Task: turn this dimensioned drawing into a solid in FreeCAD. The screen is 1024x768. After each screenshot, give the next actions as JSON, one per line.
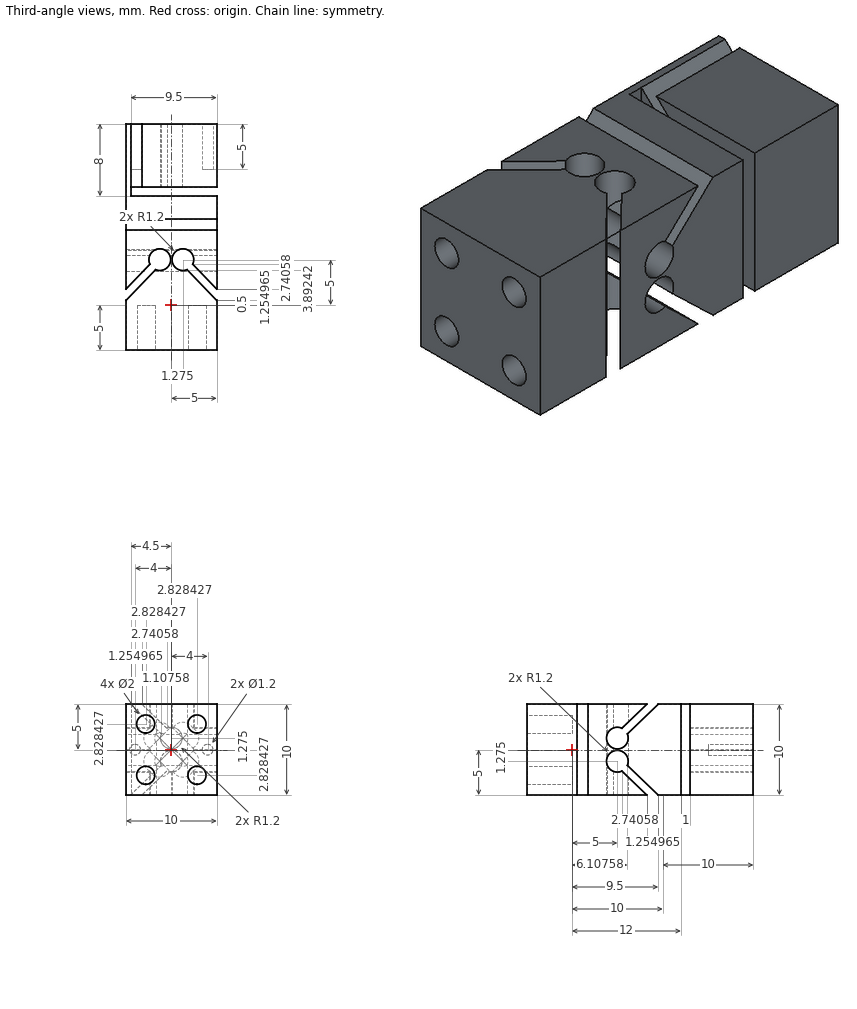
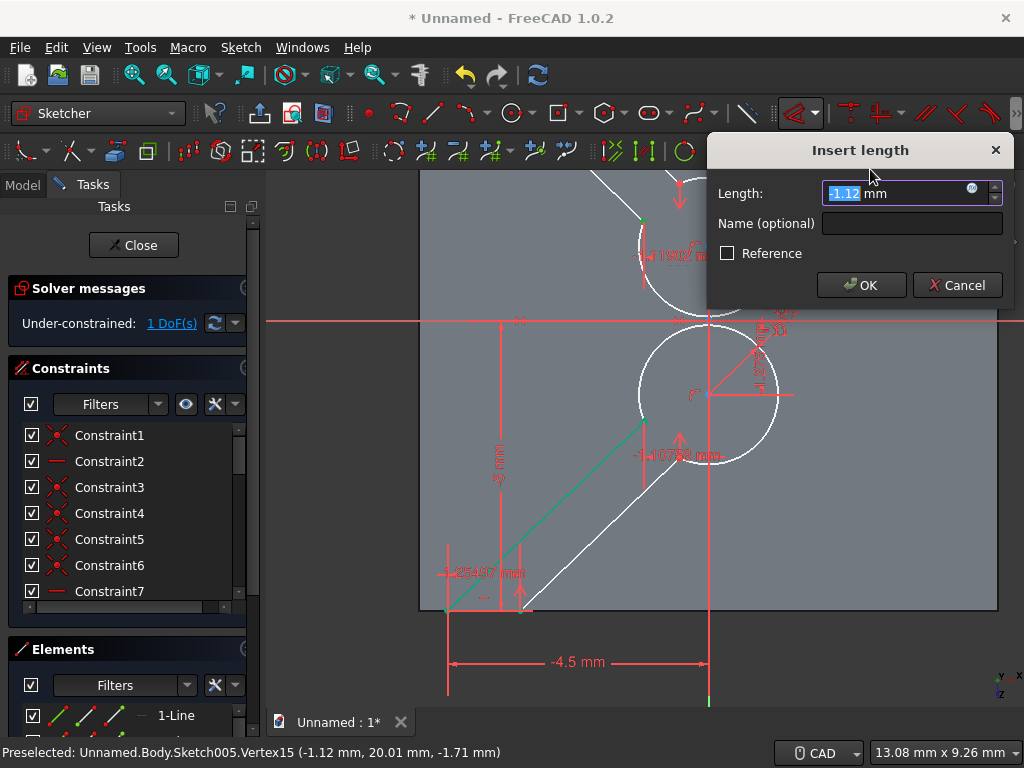
{"action": "type", "text": "-1.10758"}
{"action": "key", "text": "Return"}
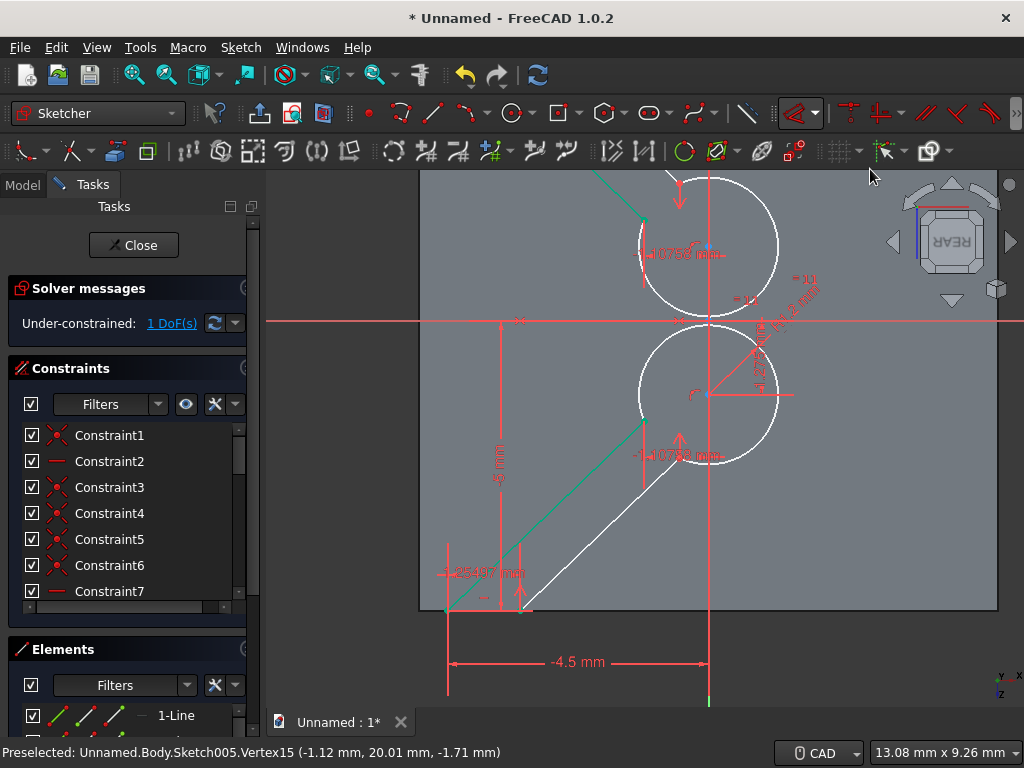
{"action": "left_click", "coordinate": [568, 565]}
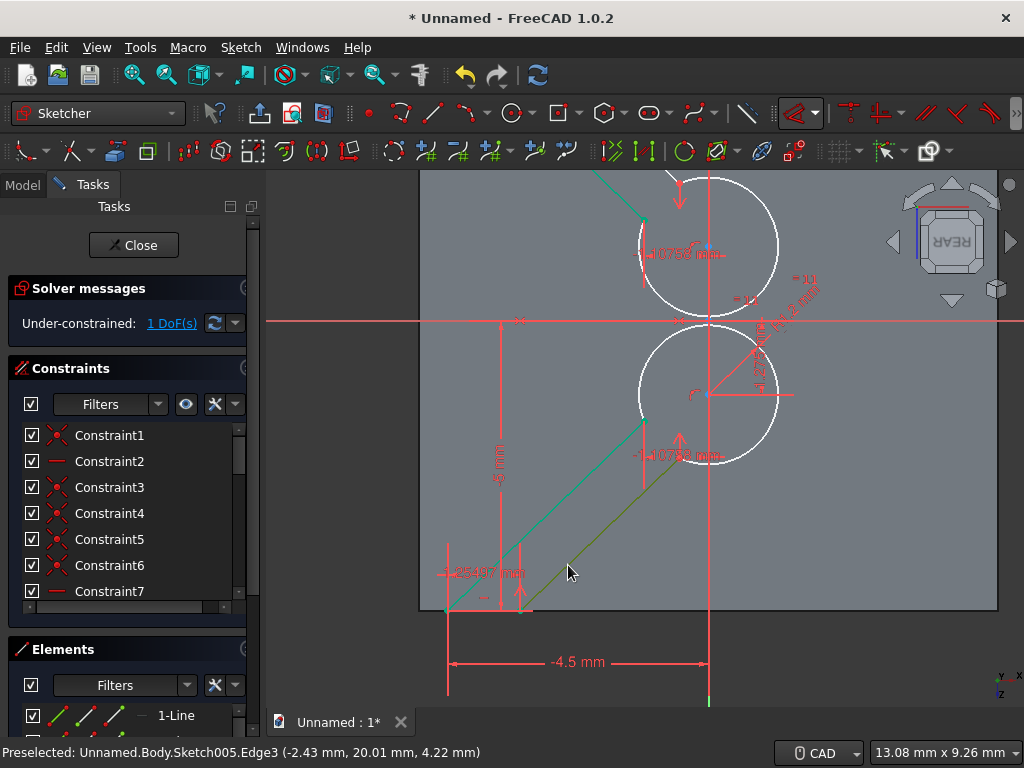
{"action": "left_click", "coordinate": [818, 114]}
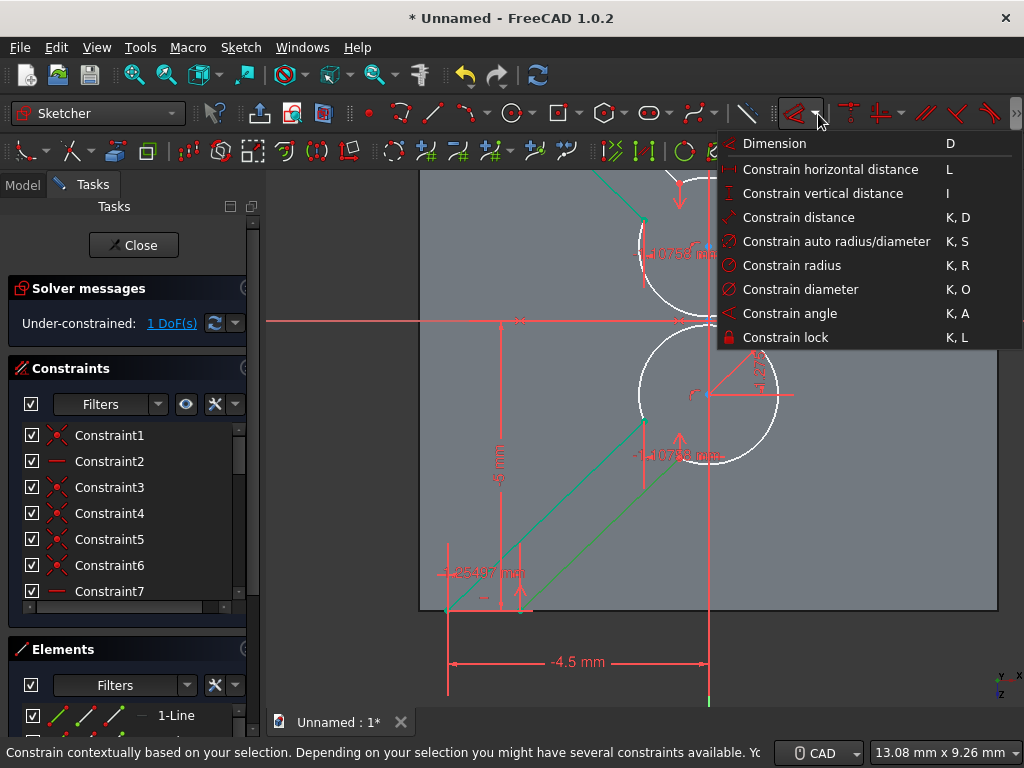
{"action": "left_click", "coordinate": [870, 169]}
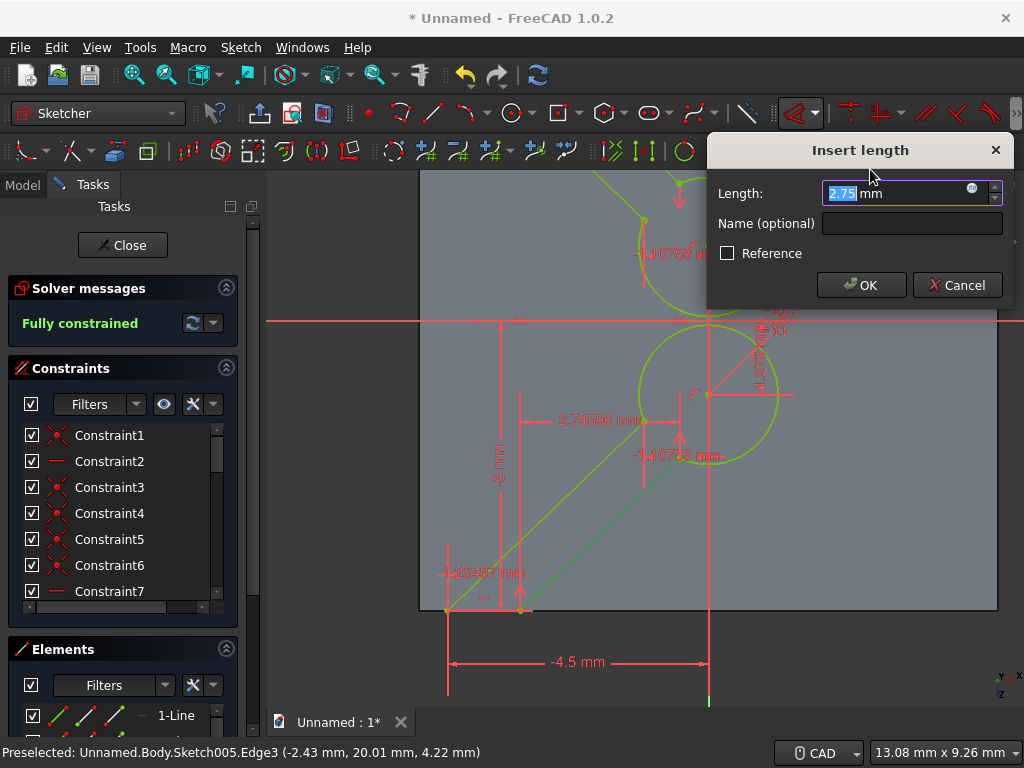
{"action": "type", "text": "2.74058"}
{"action": "key", "text": "Return"}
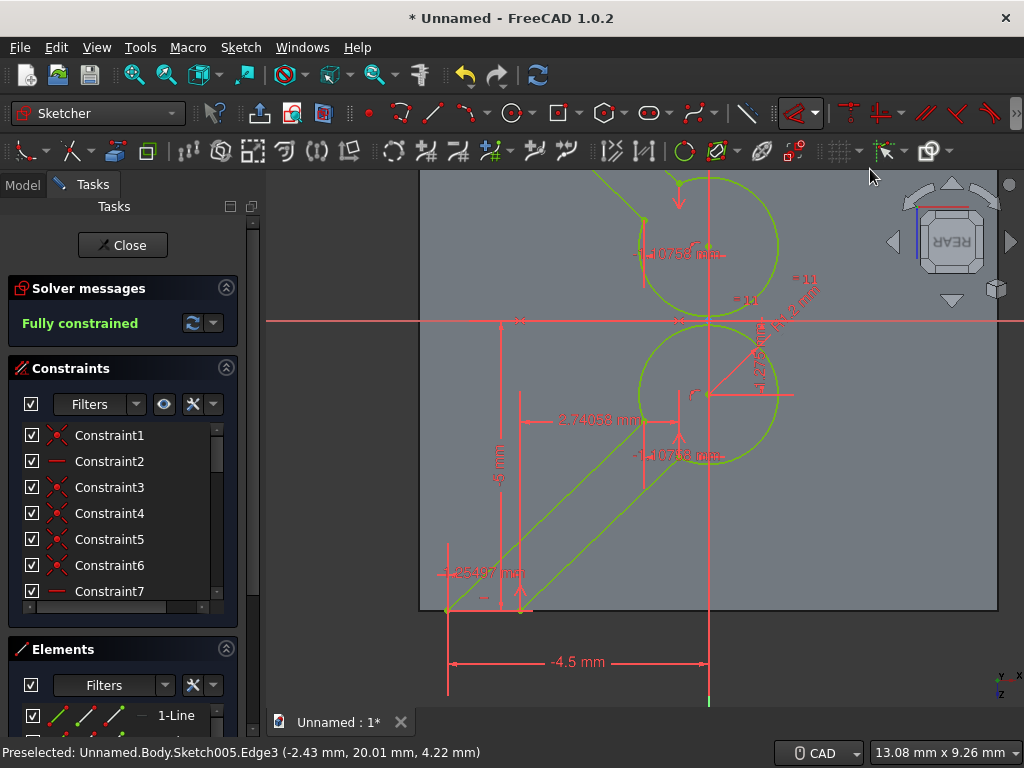
{"action": "left_click", "coordinate": [123, 245]}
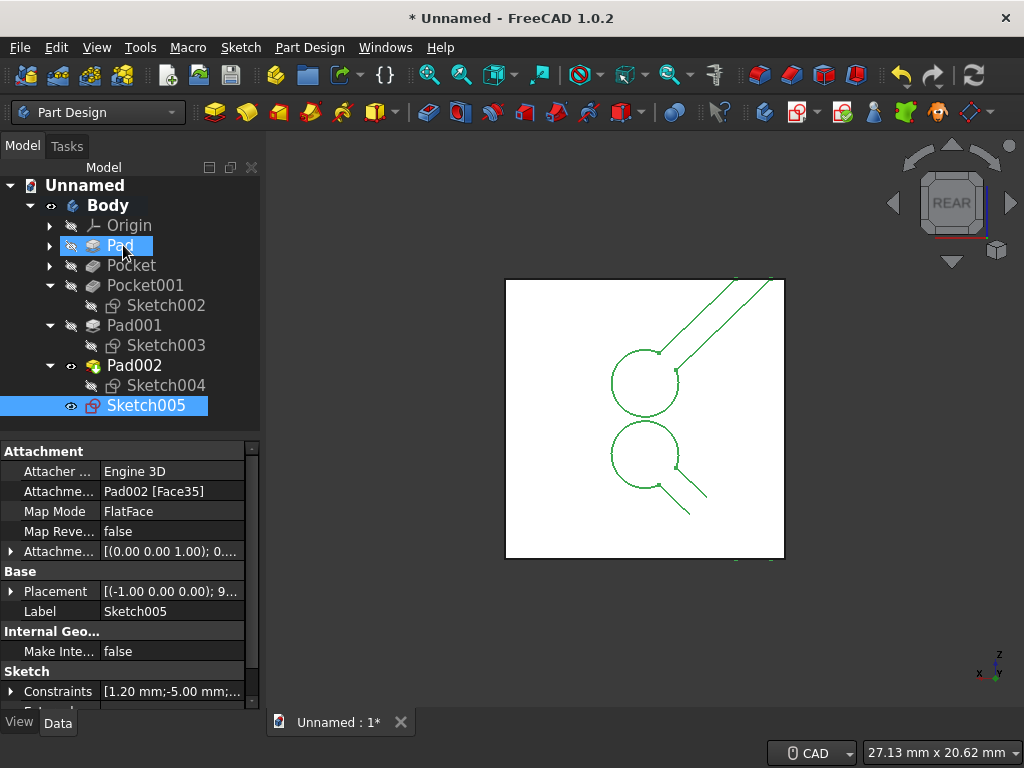
{"action": "left_click", "coordinate": [430, 112]}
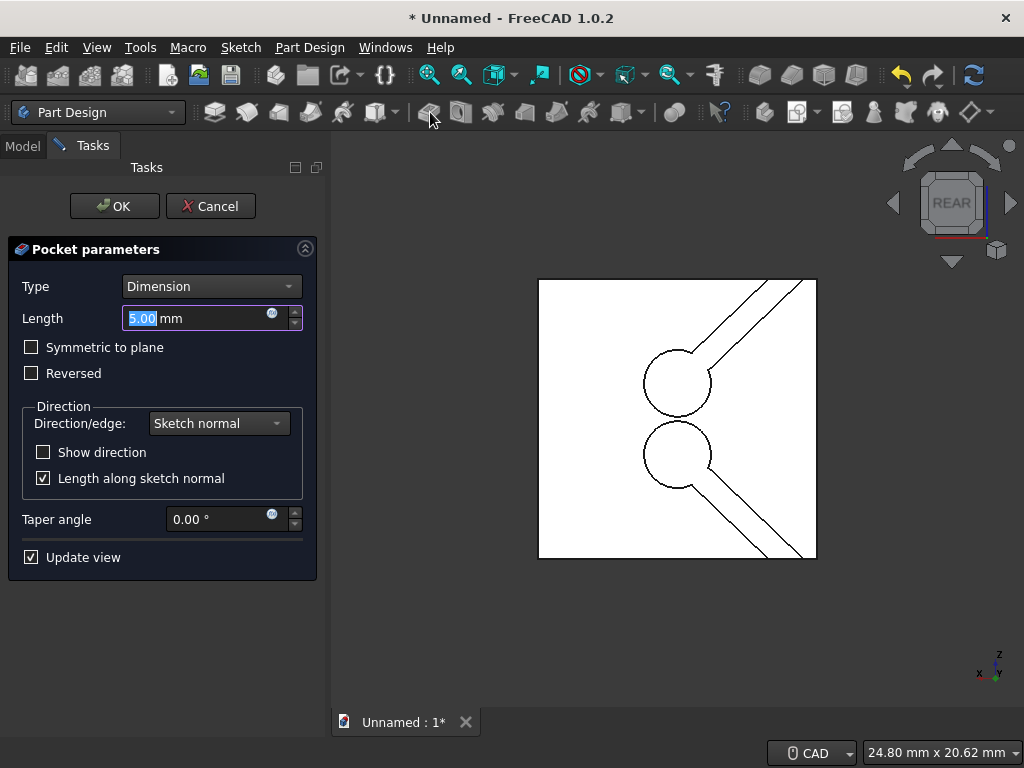
{"action": "type", "text": "8"}
{"action": "key", "text": "Tab"}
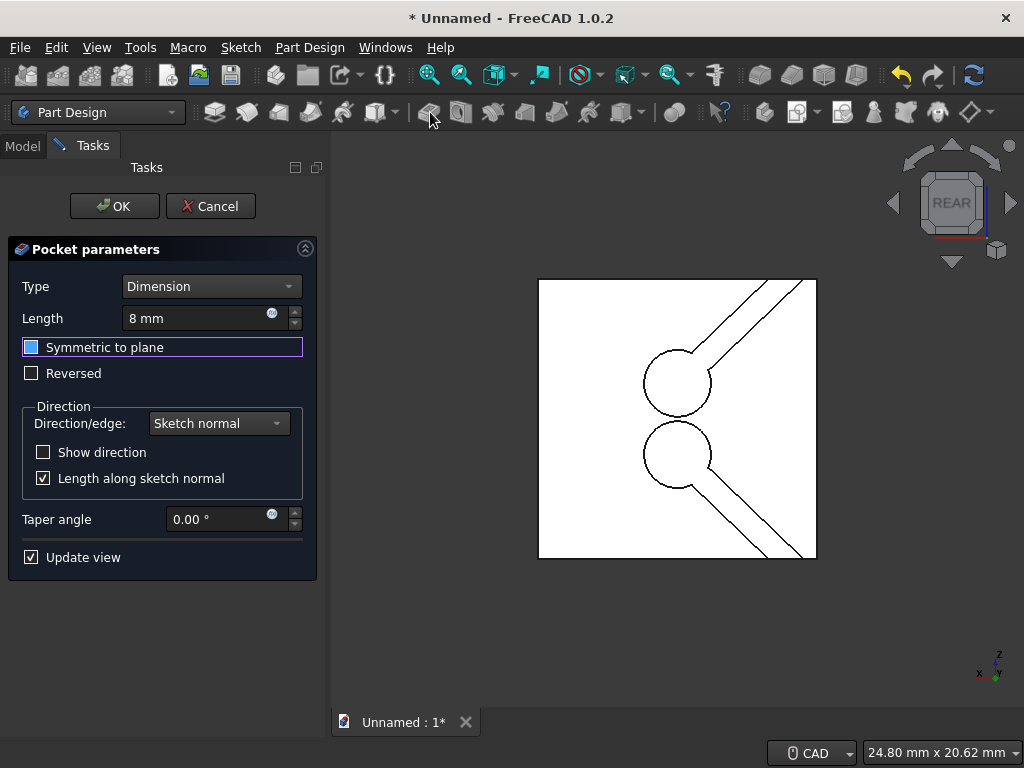
{"action": "left_click", "coordinate": [115, 206]}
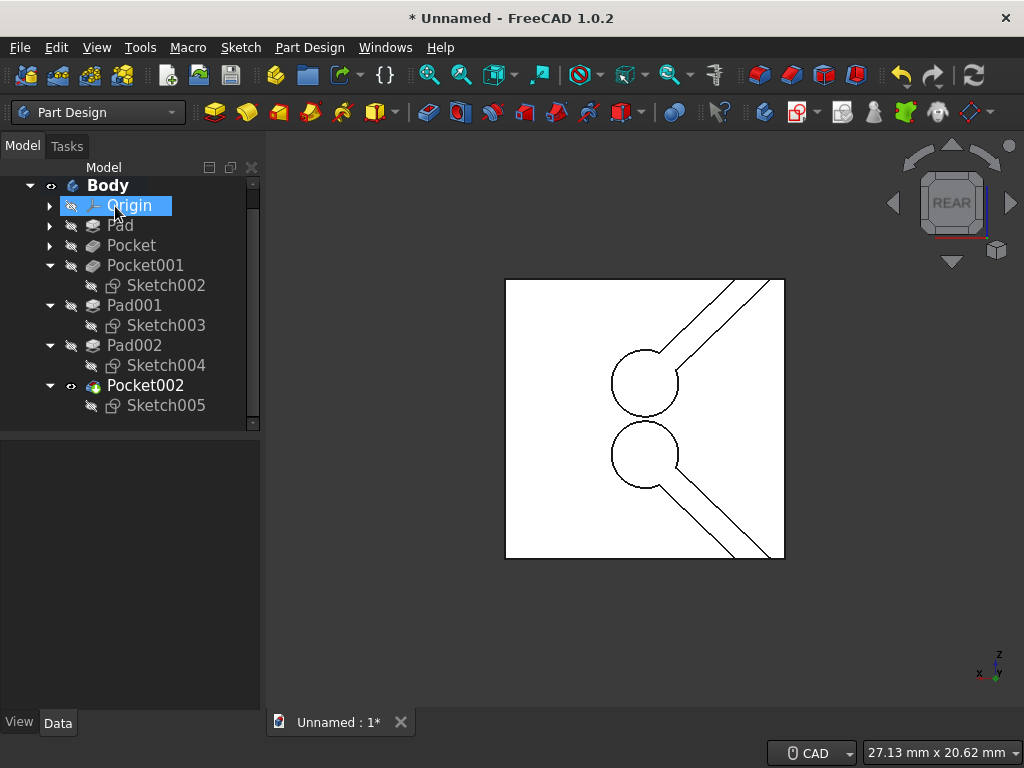
{"action": "key", "text": "0"}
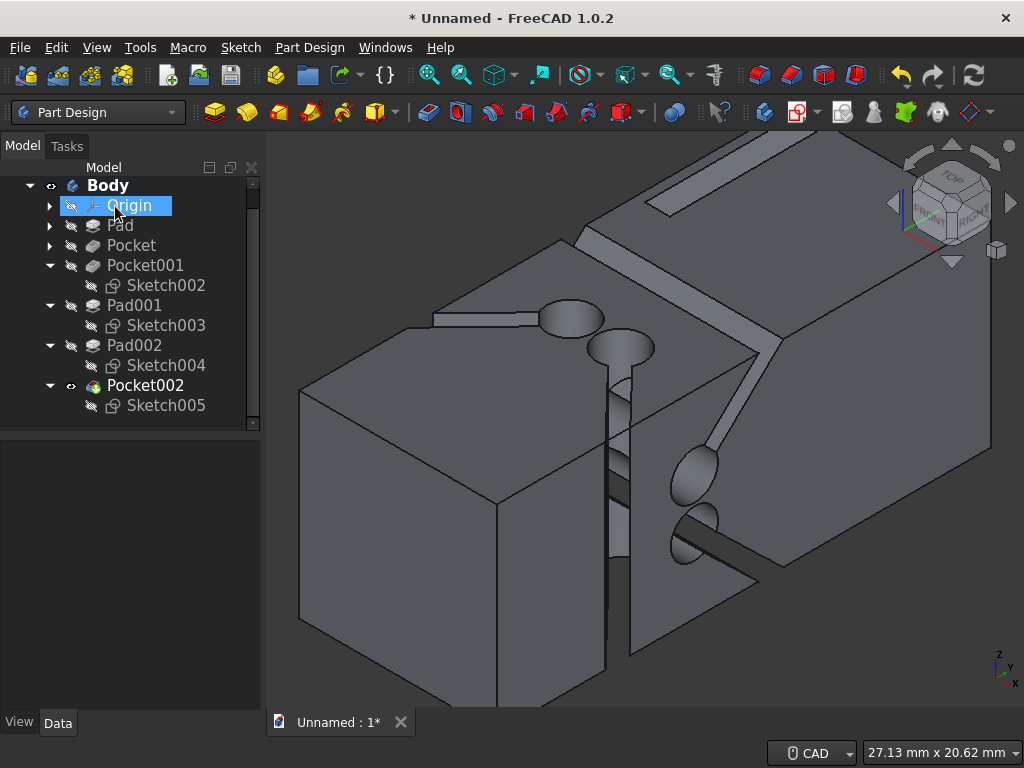
{"action": "left_click", "coordinate": [430, 76]}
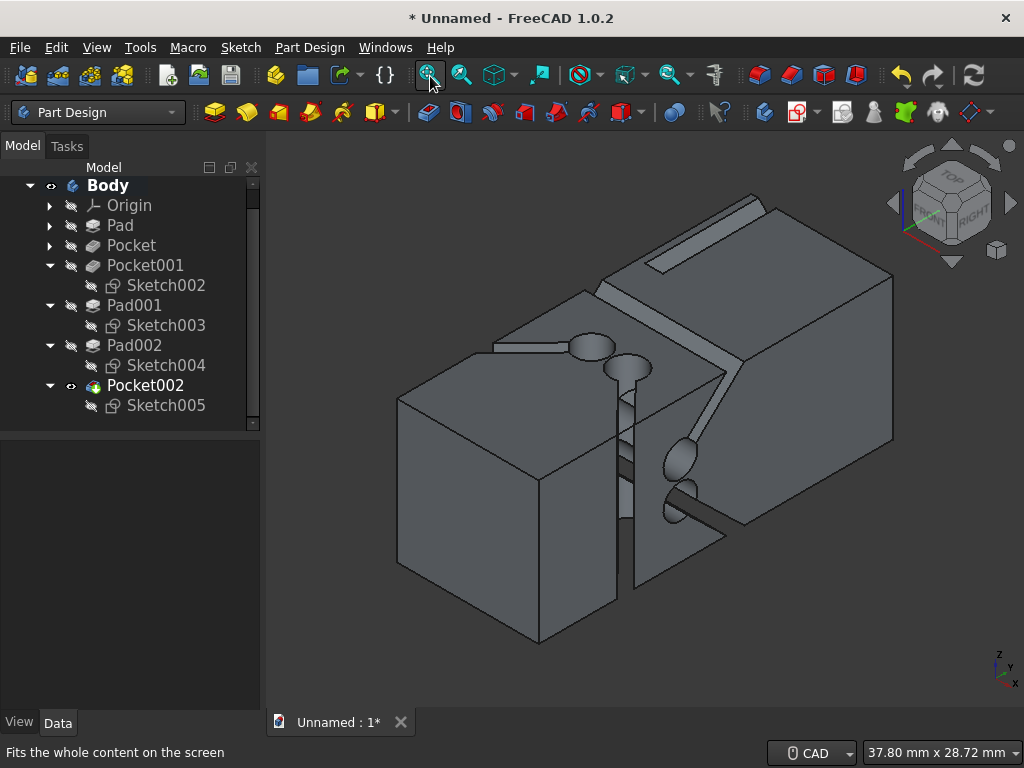
{"action": "left_click", "coordinate": [801, 410]}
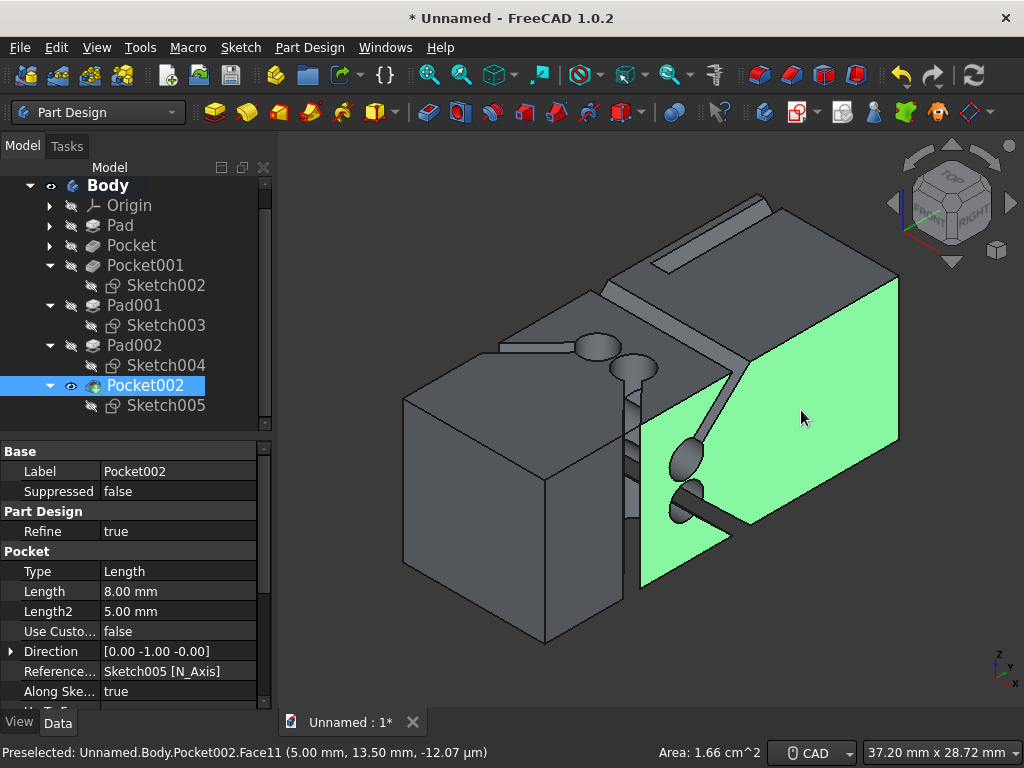
{"action": "left_click", "coordinate": [798, 112]}